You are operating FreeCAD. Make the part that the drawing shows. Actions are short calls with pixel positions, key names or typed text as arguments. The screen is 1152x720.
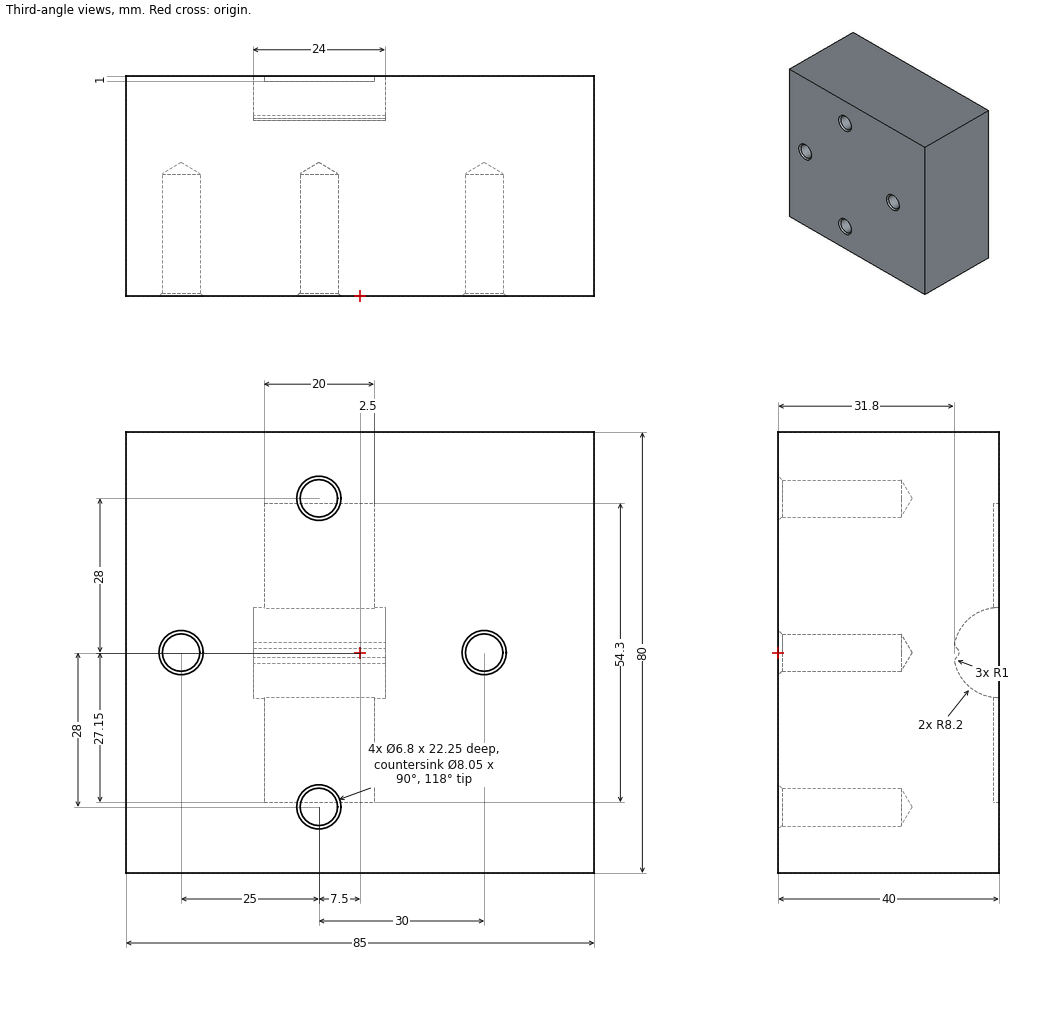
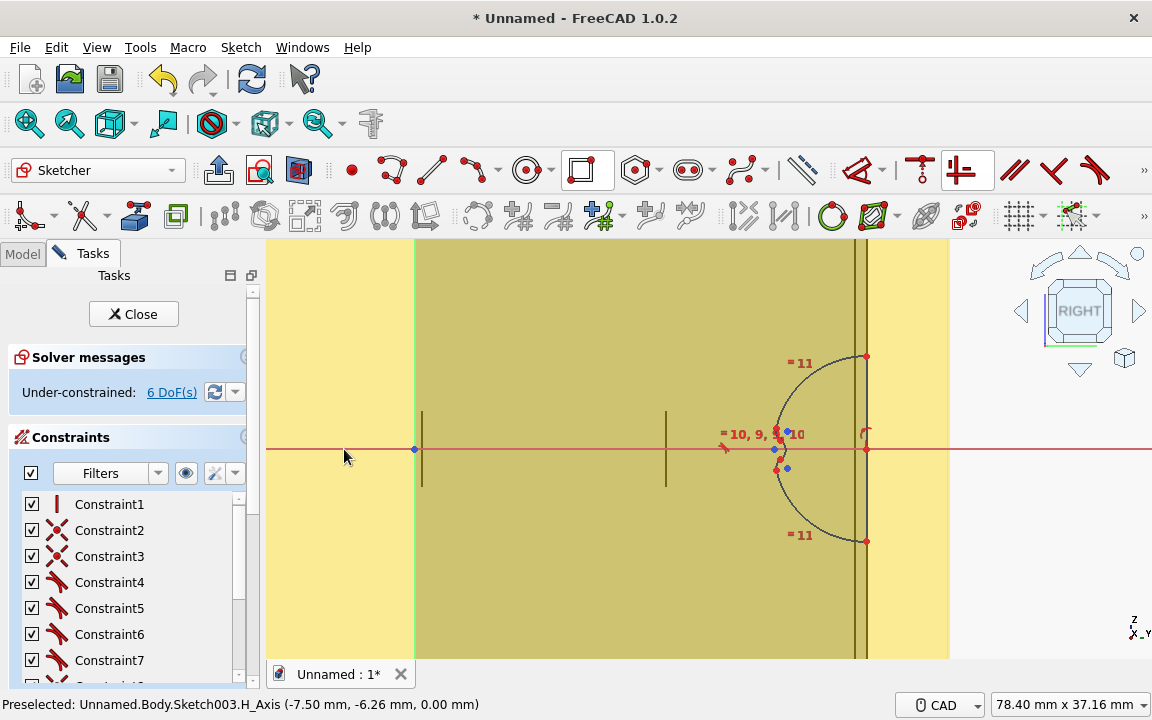
scroll(774, 450, up, 4)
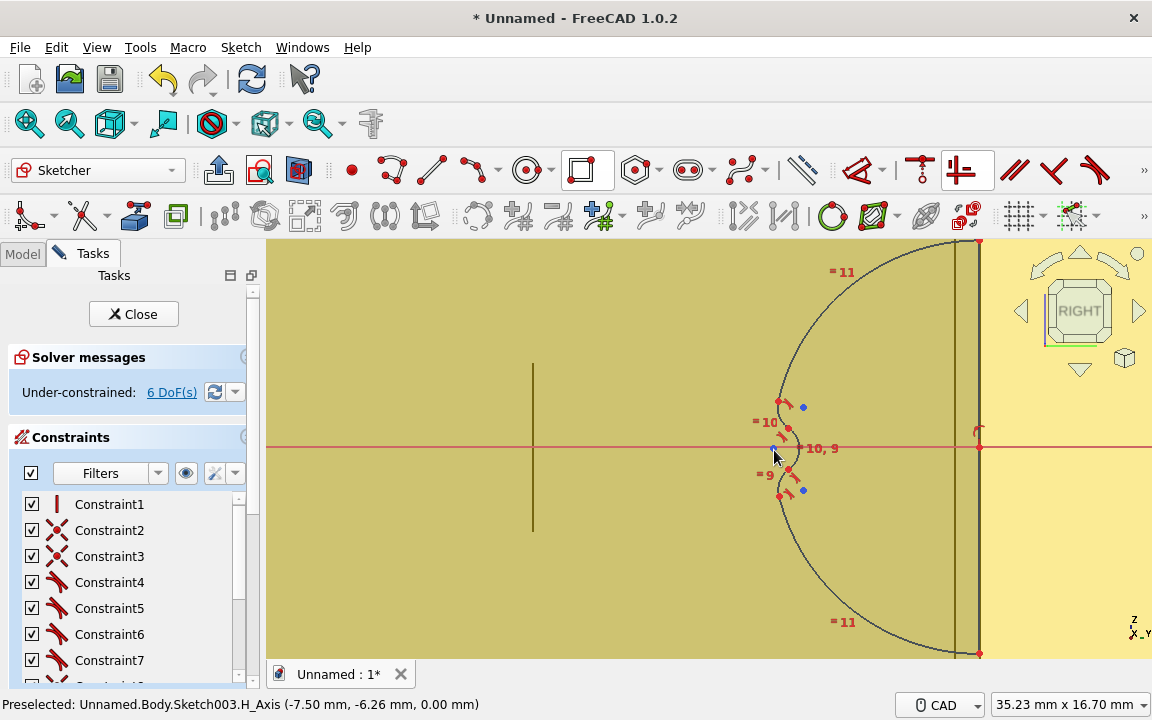
click(774, 449)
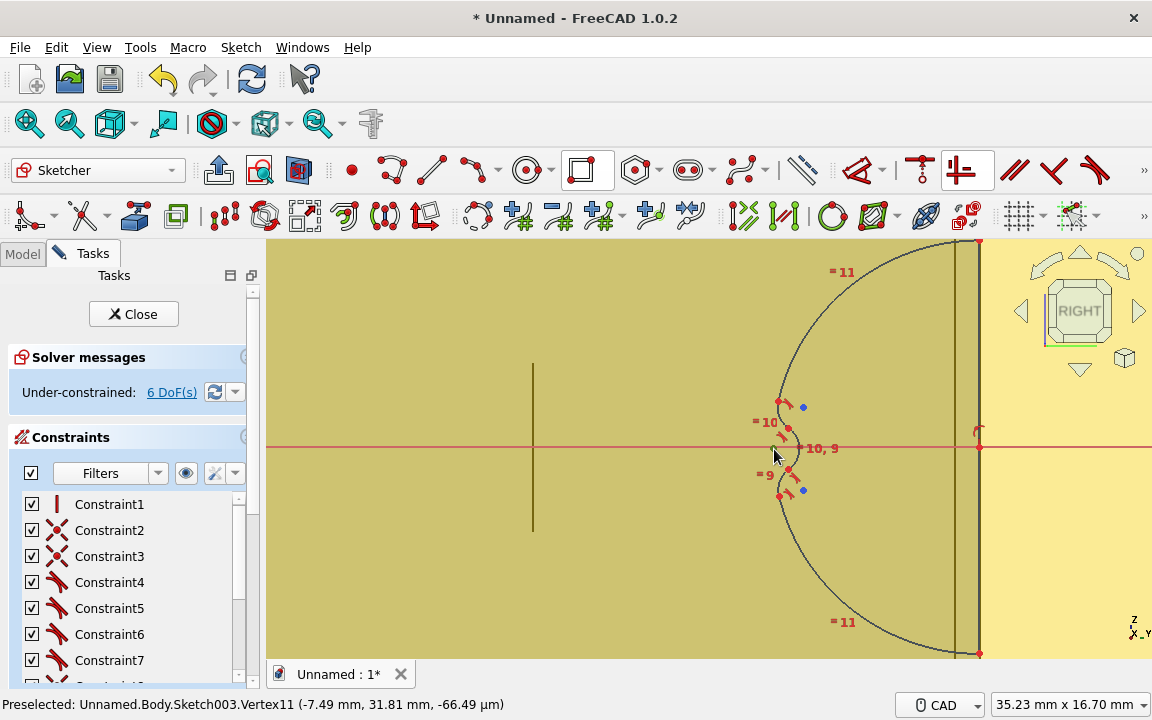
click(344, 447)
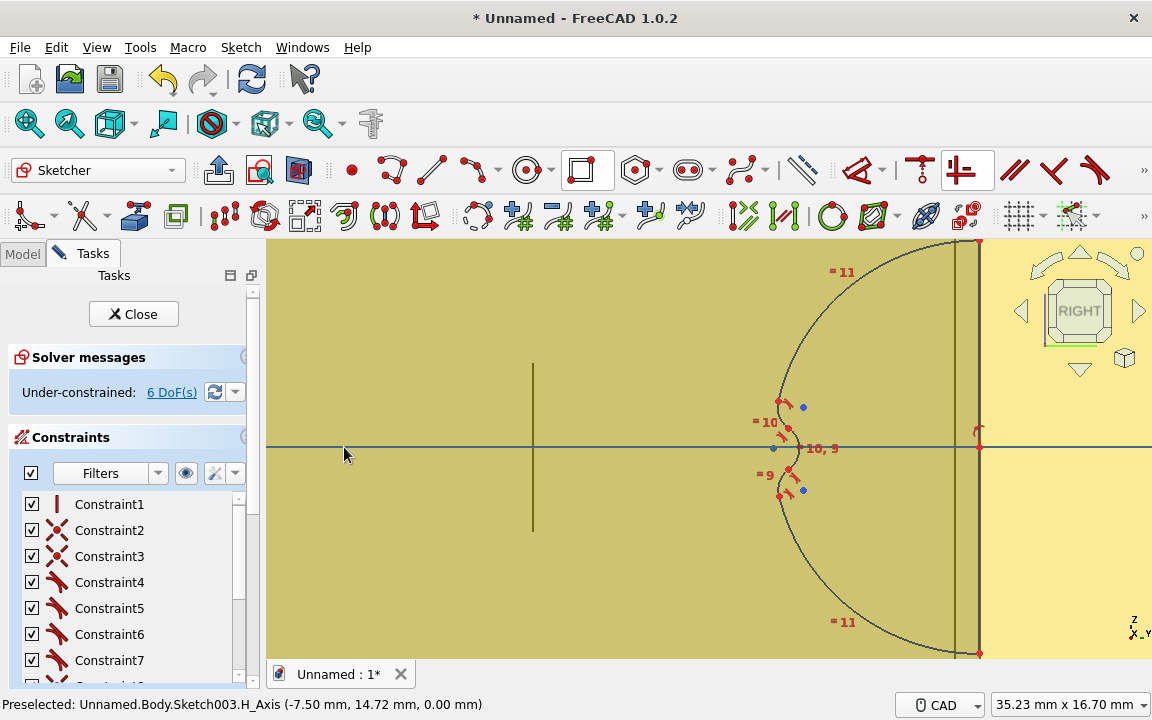
click(920, 170)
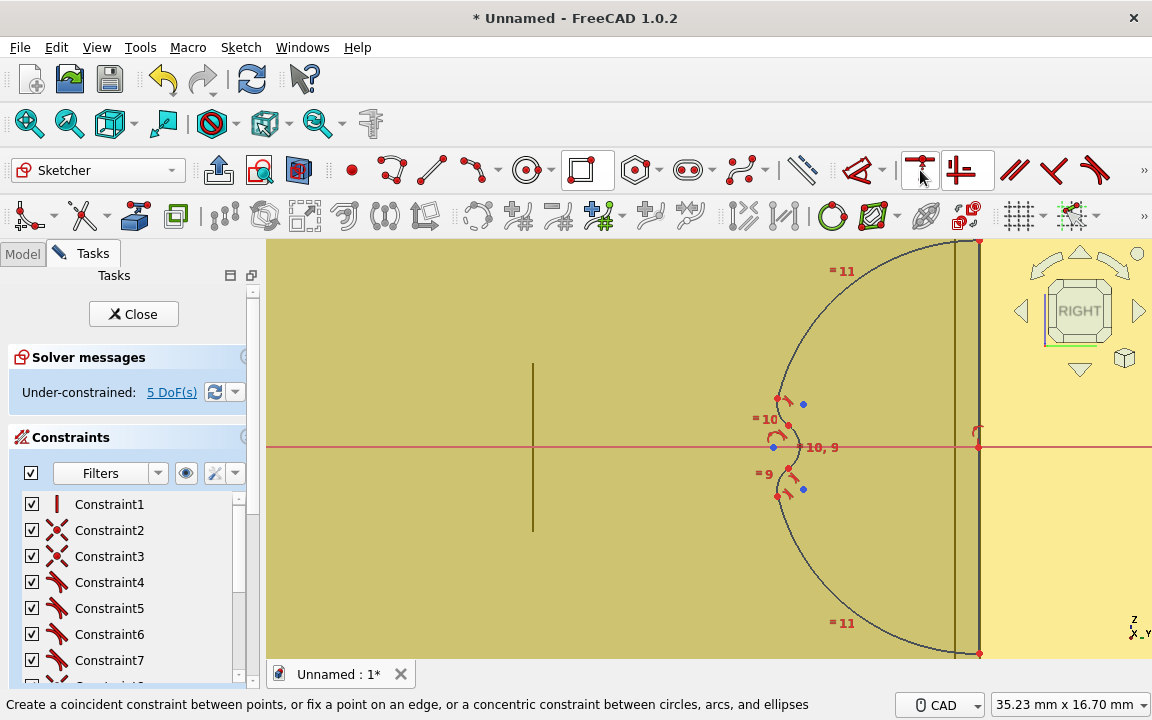
click(858, 170)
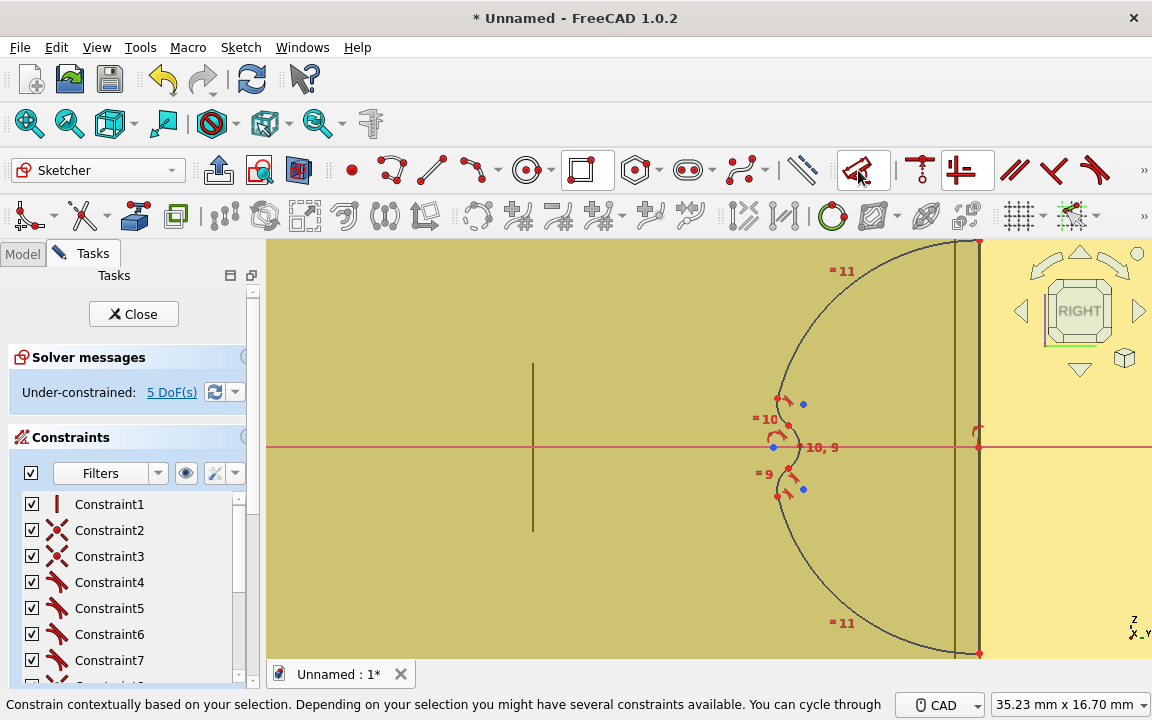
click(813, 571)
click(787, 590)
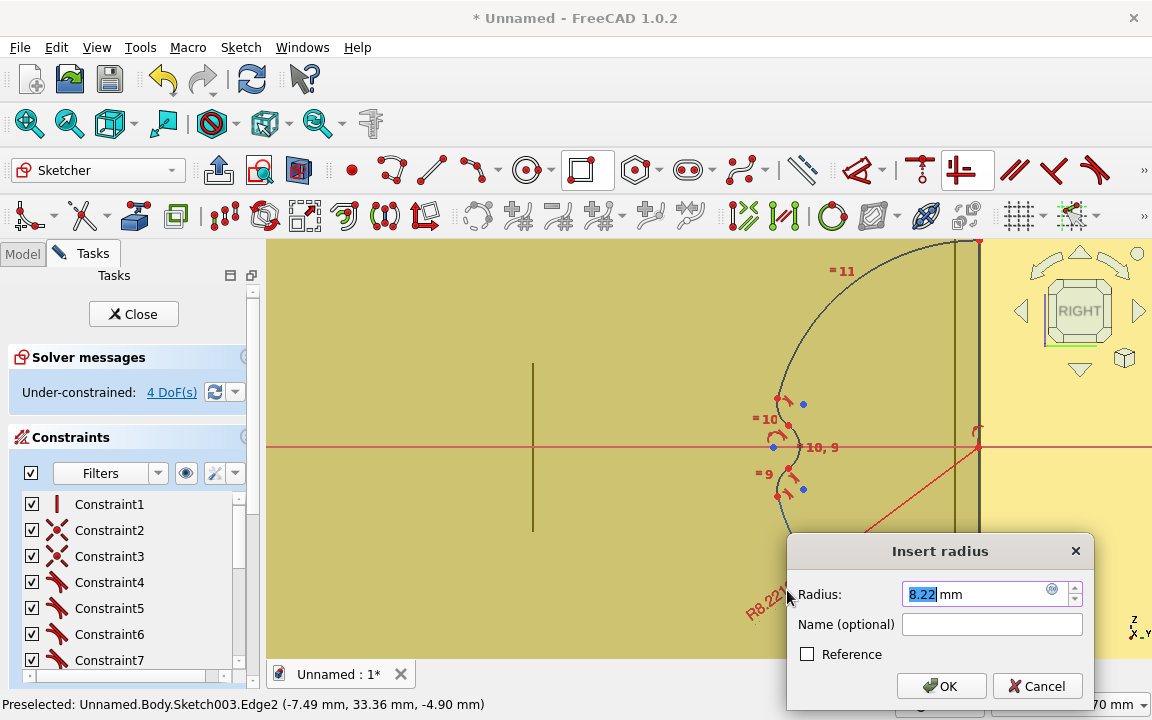
text(8.2)
key(Return)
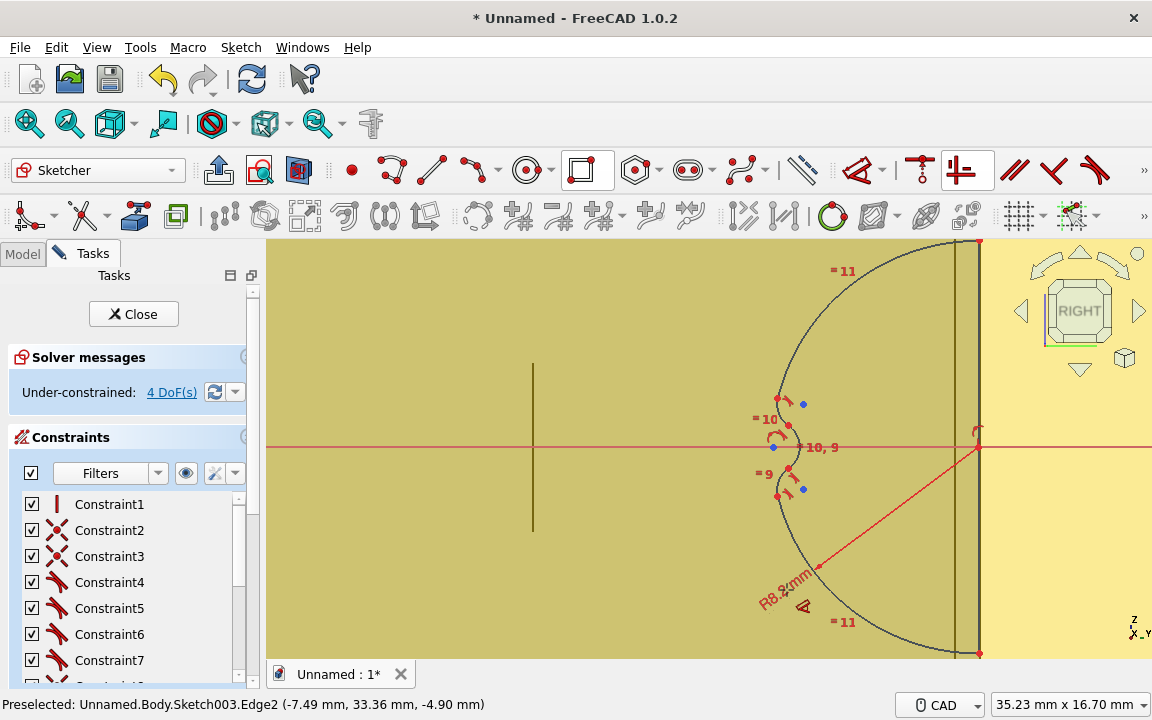
scroll(782, 475, up, 3)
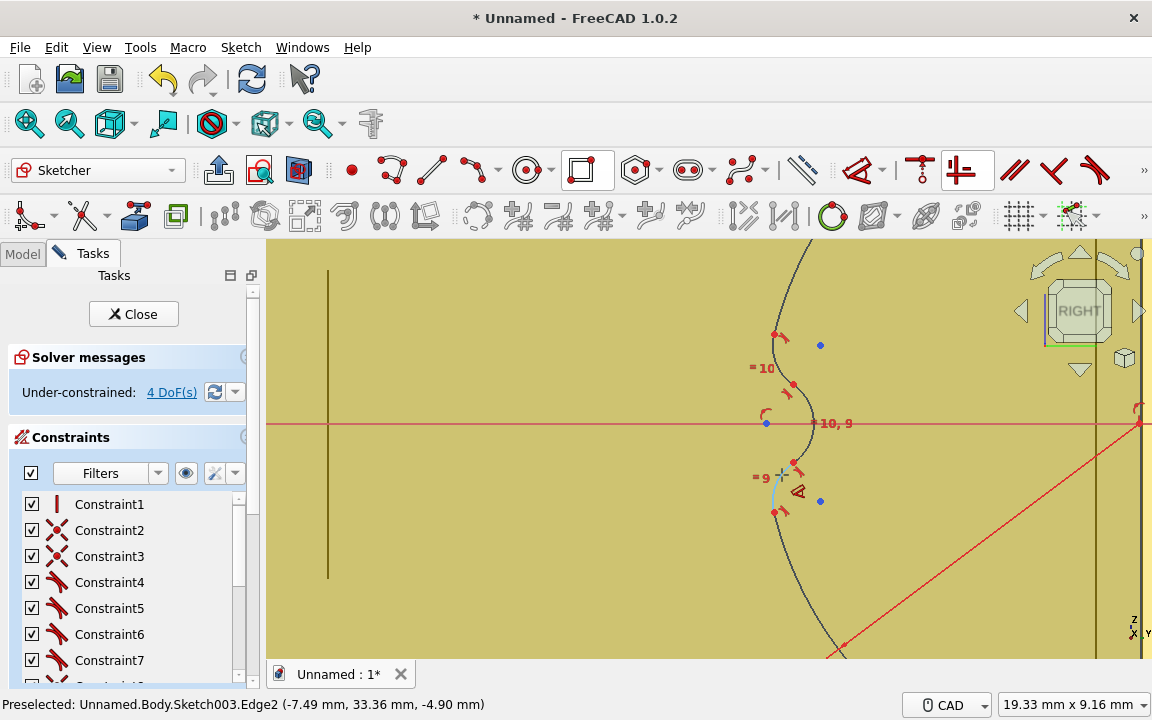
click(781, 475)
click(755, 457)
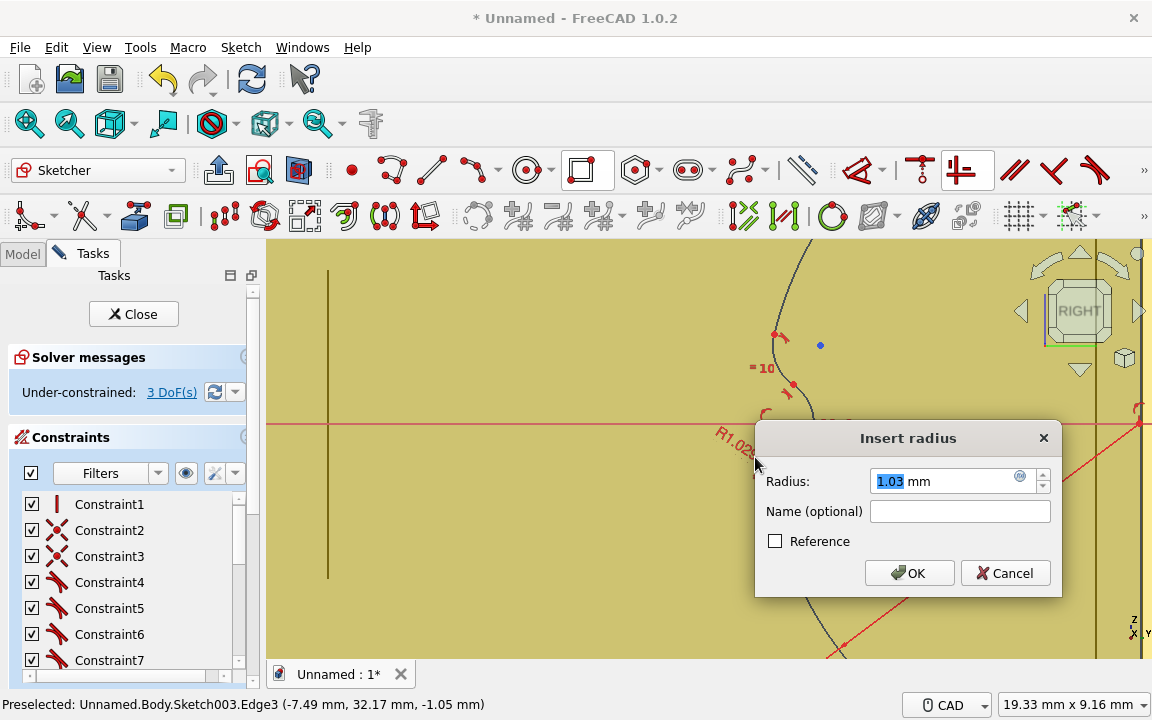
text(1)
key(Return)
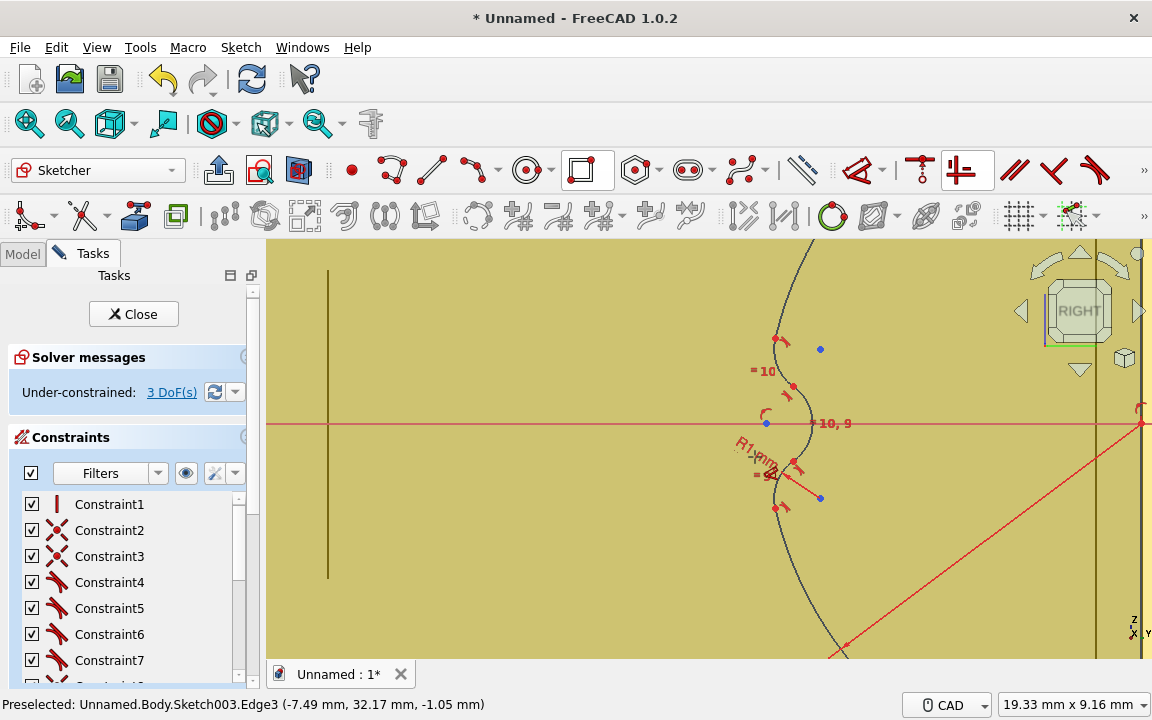
scroll(776, 457, down, 7)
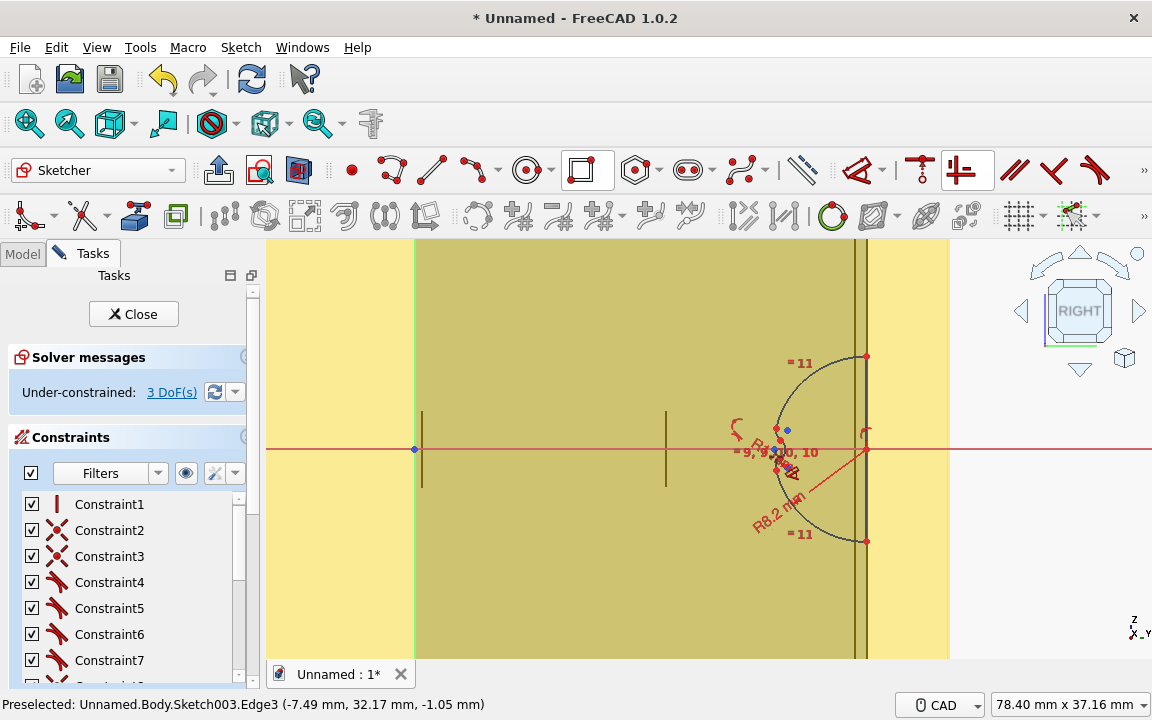
click(866, 357)
click(641, 323)